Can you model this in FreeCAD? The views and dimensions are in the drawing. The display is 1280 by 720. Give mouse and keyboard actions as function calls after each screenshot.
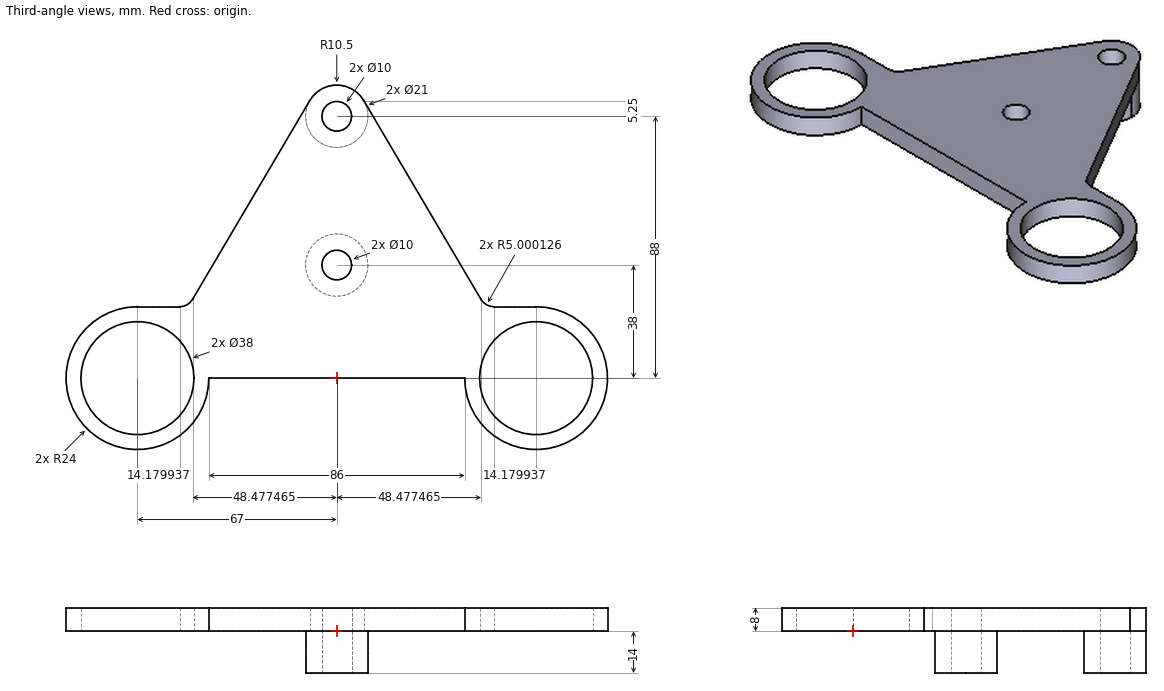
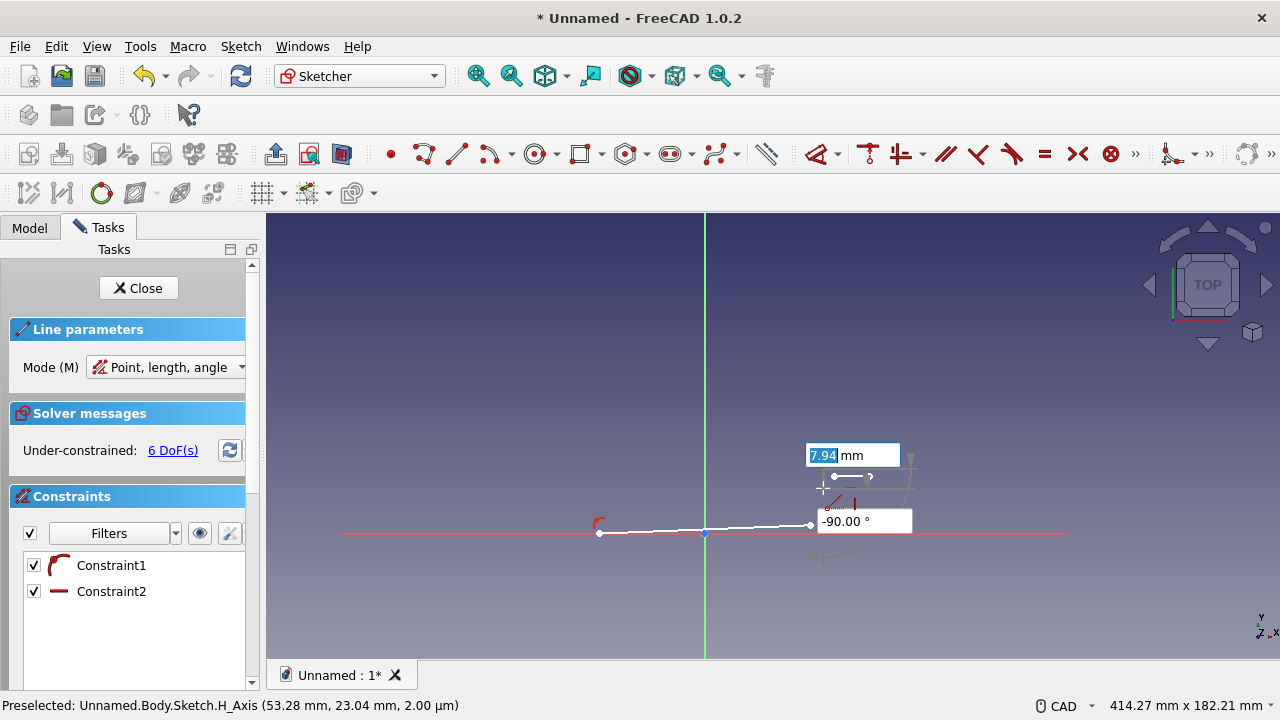
click(727, 305)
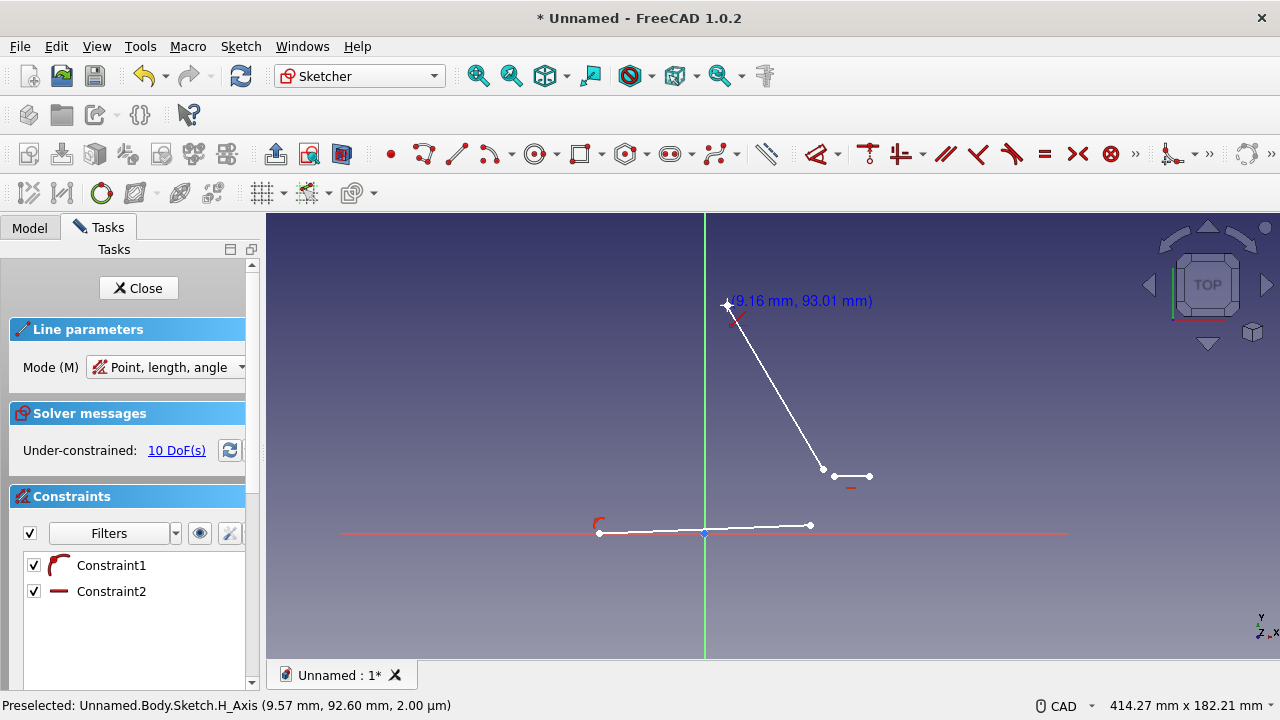
click(682, 305)
click(586, 469)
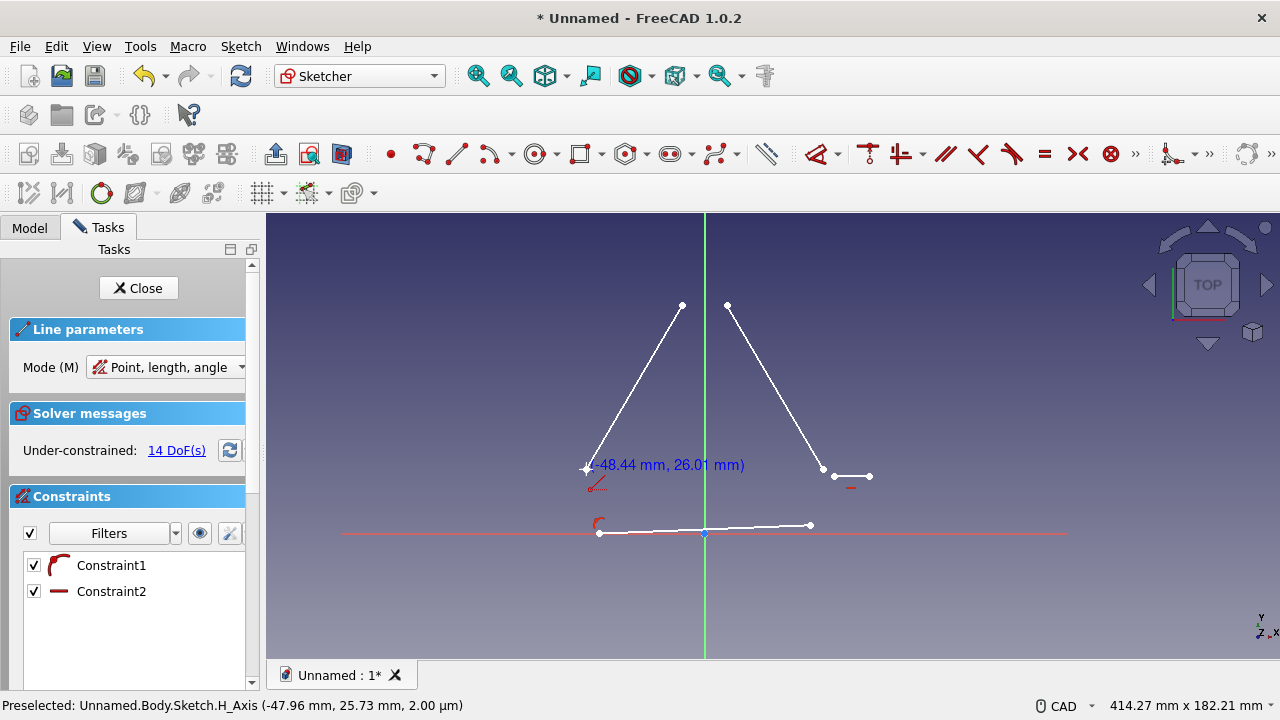
scroll(575, 475, up, 2)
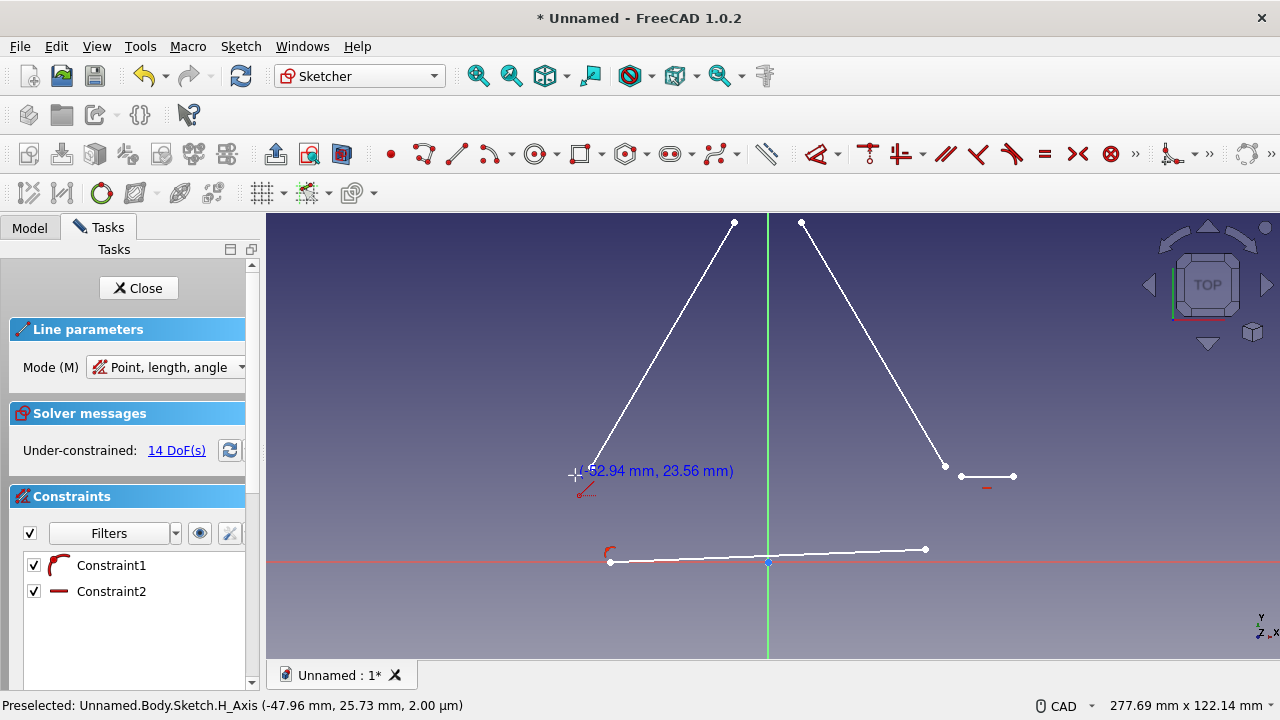
click(575, 475)
click(524, 475)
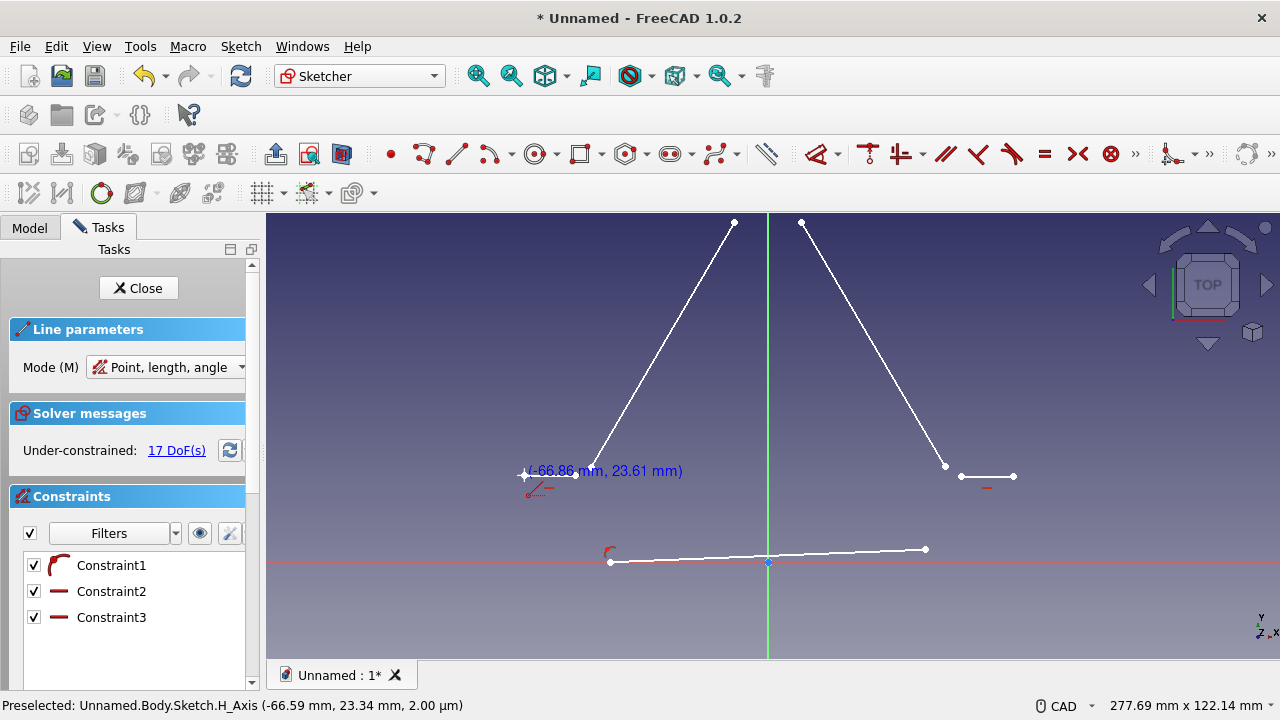
key(g)
key(3)
key(a)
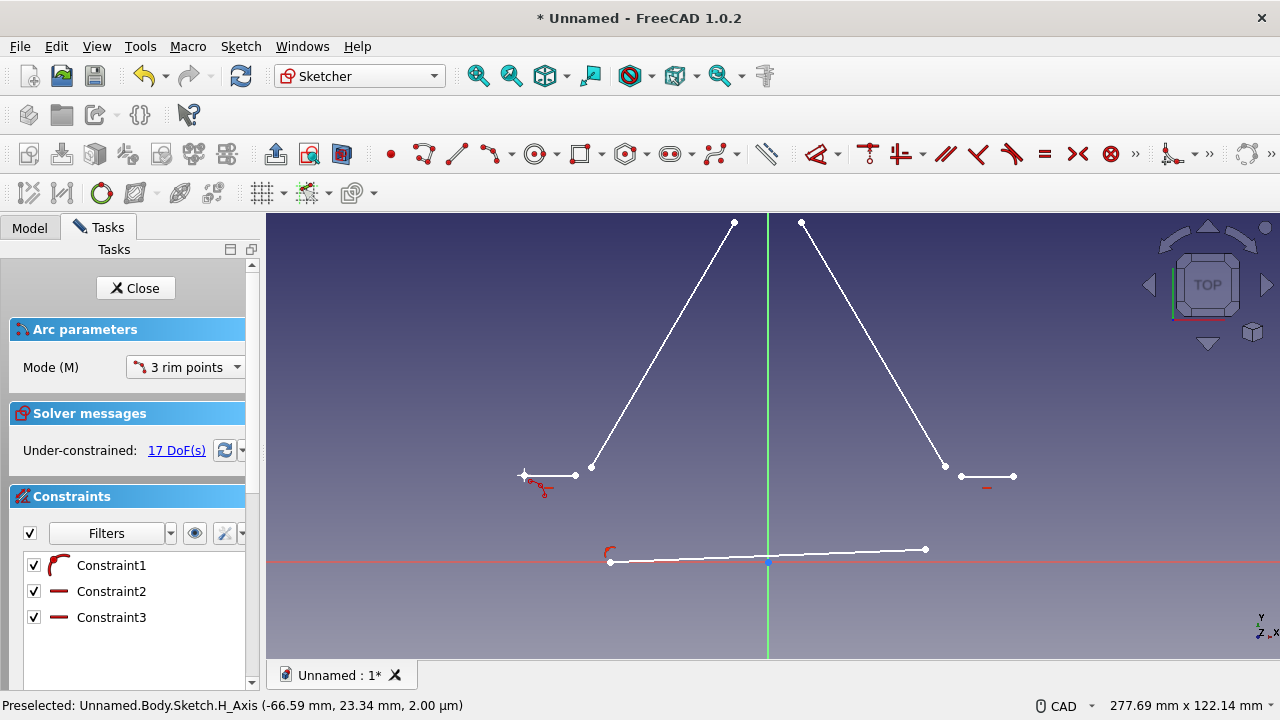
click(925, 550)
click(1013, 477)
click(1075, 624)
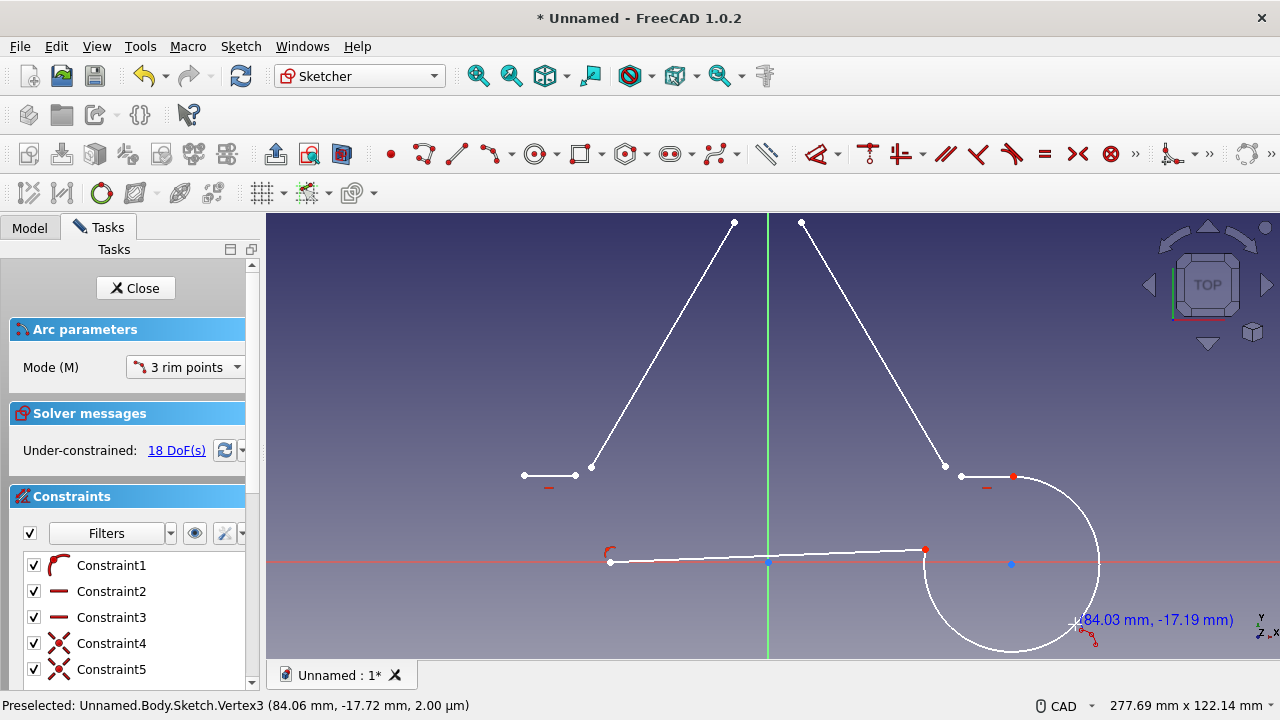
click(961, 477)
click(945, 466)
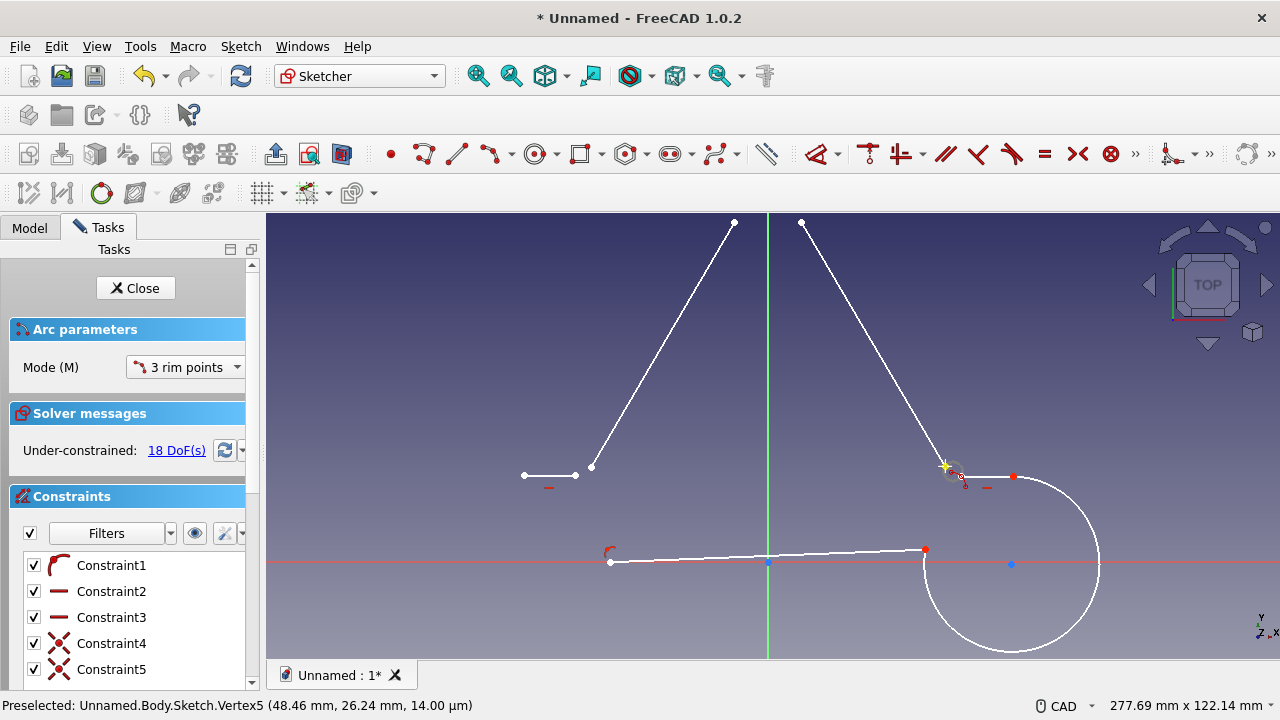
scroll(952, 472, up, 10)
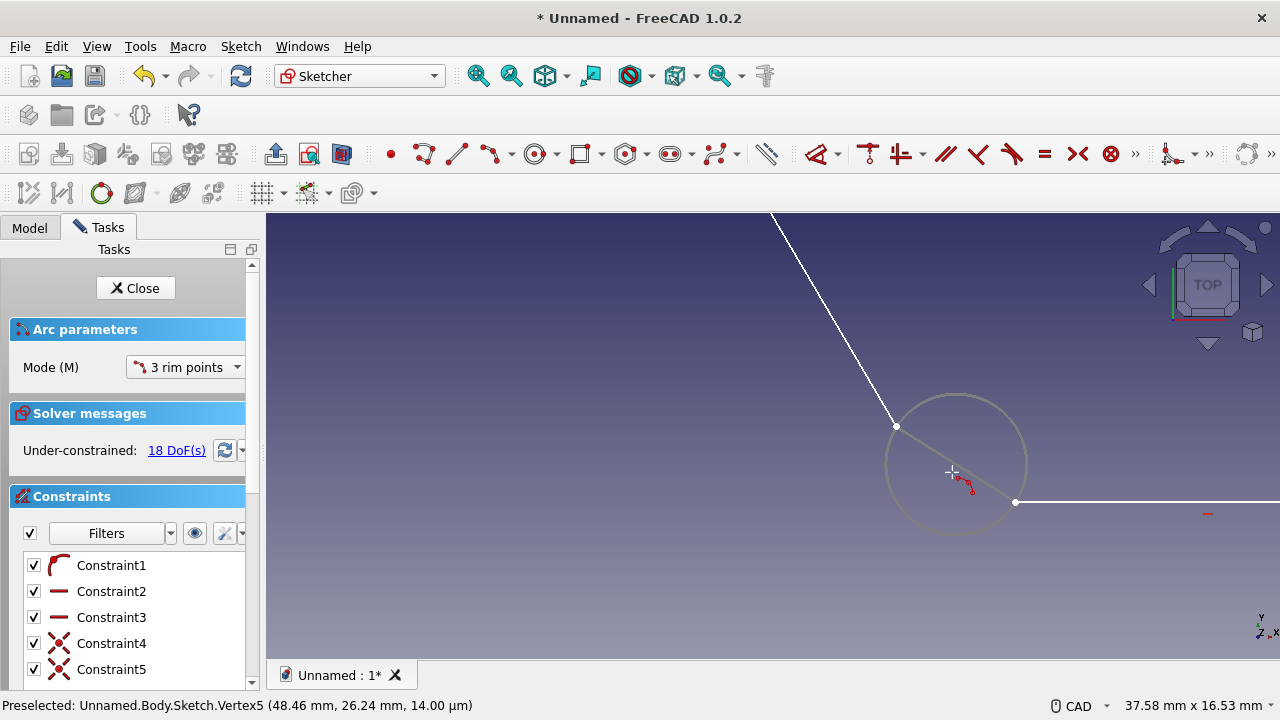
click(947, 470)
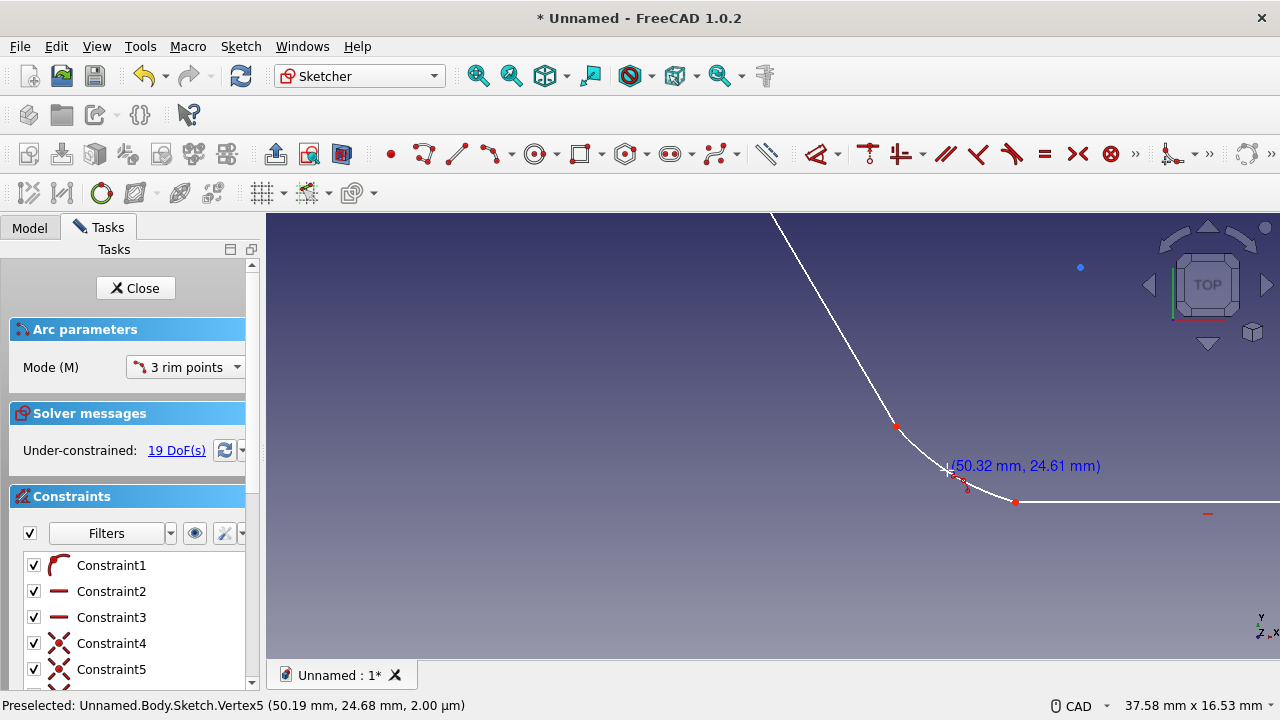
scroll(816, 473, down, 12)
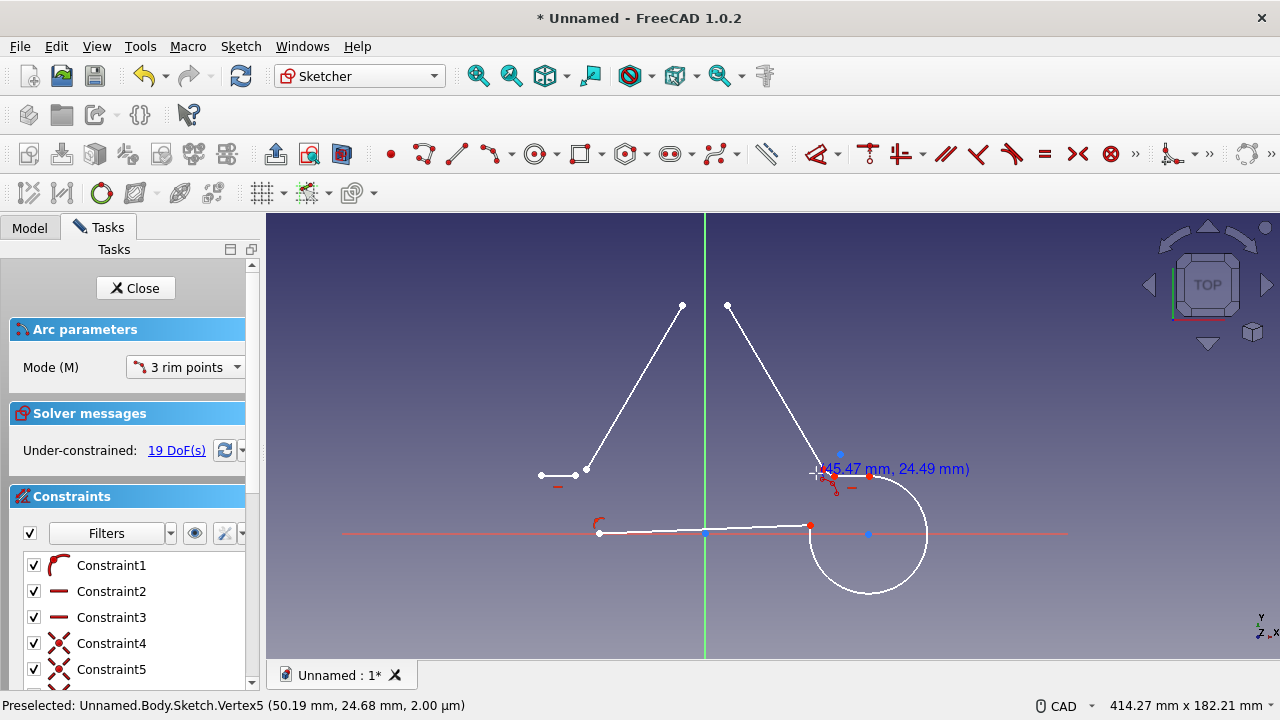
click(728, 306)
click(683, 306)